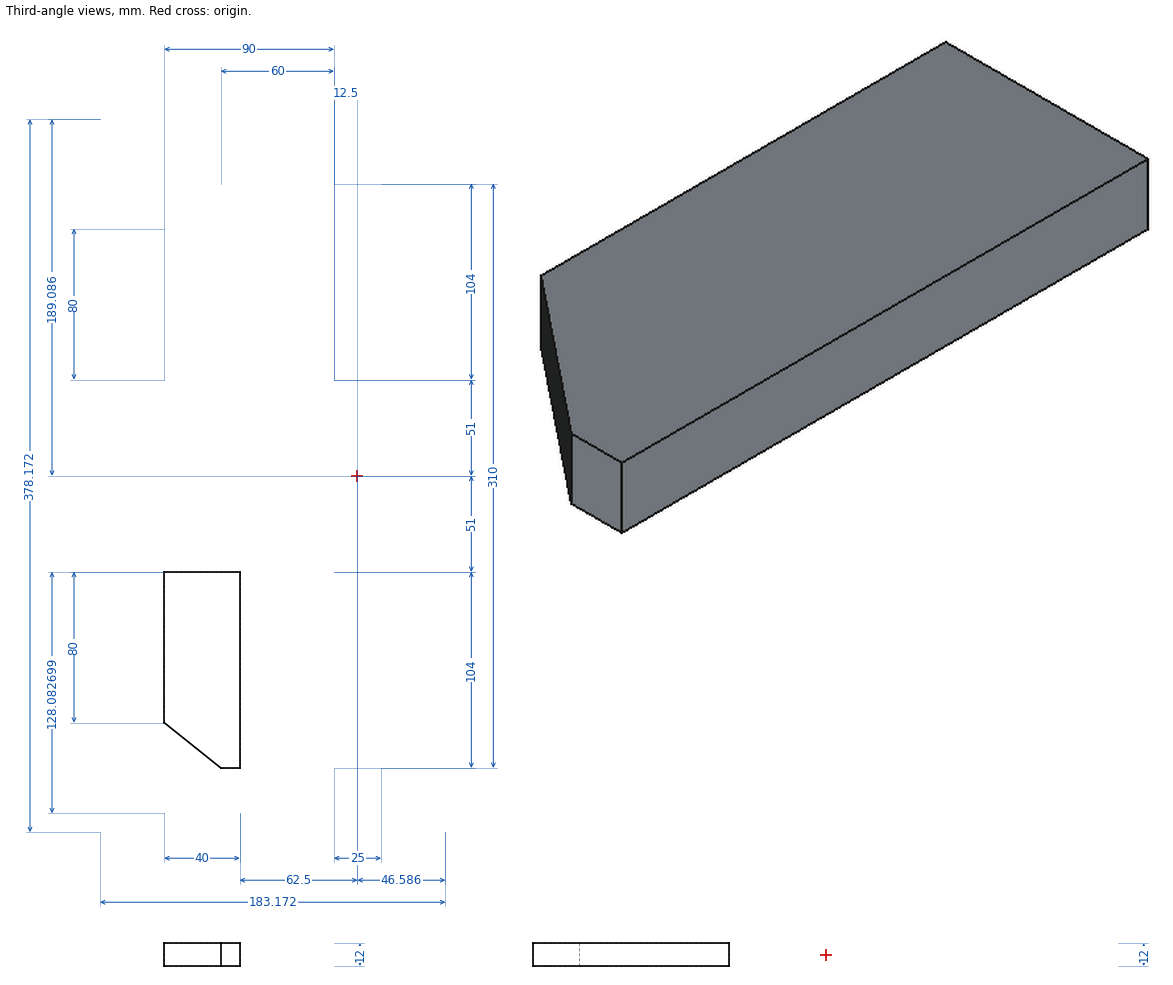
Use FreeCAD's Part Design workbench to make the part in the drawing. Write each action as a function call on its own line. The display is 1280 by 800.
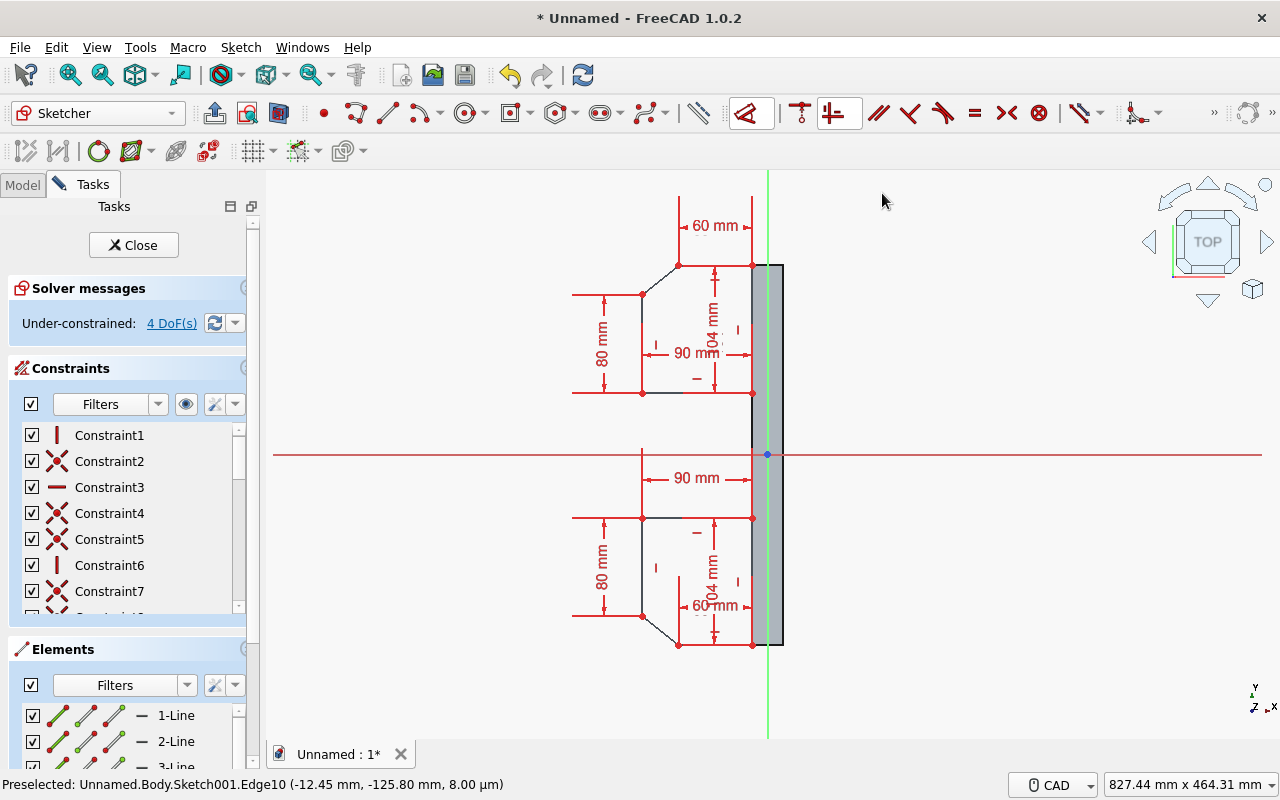
click(752, 393)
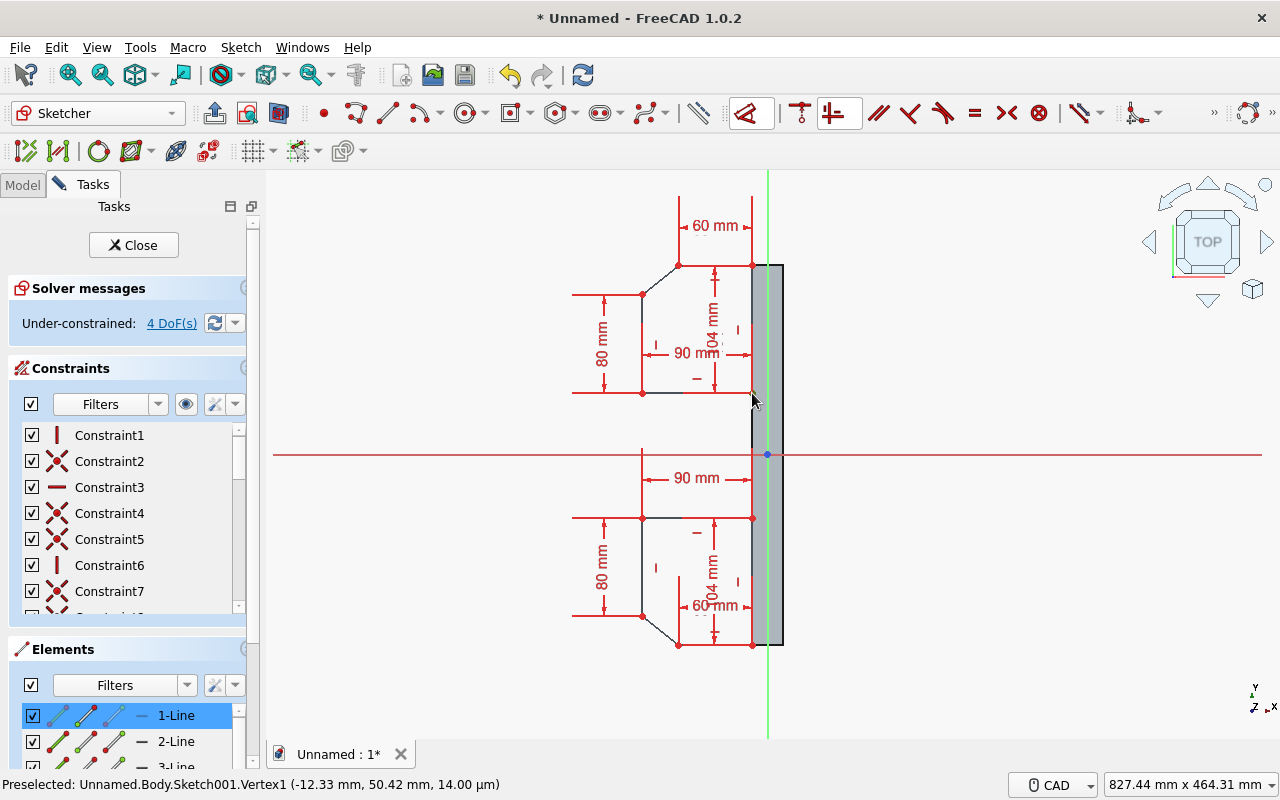
click(768, 114)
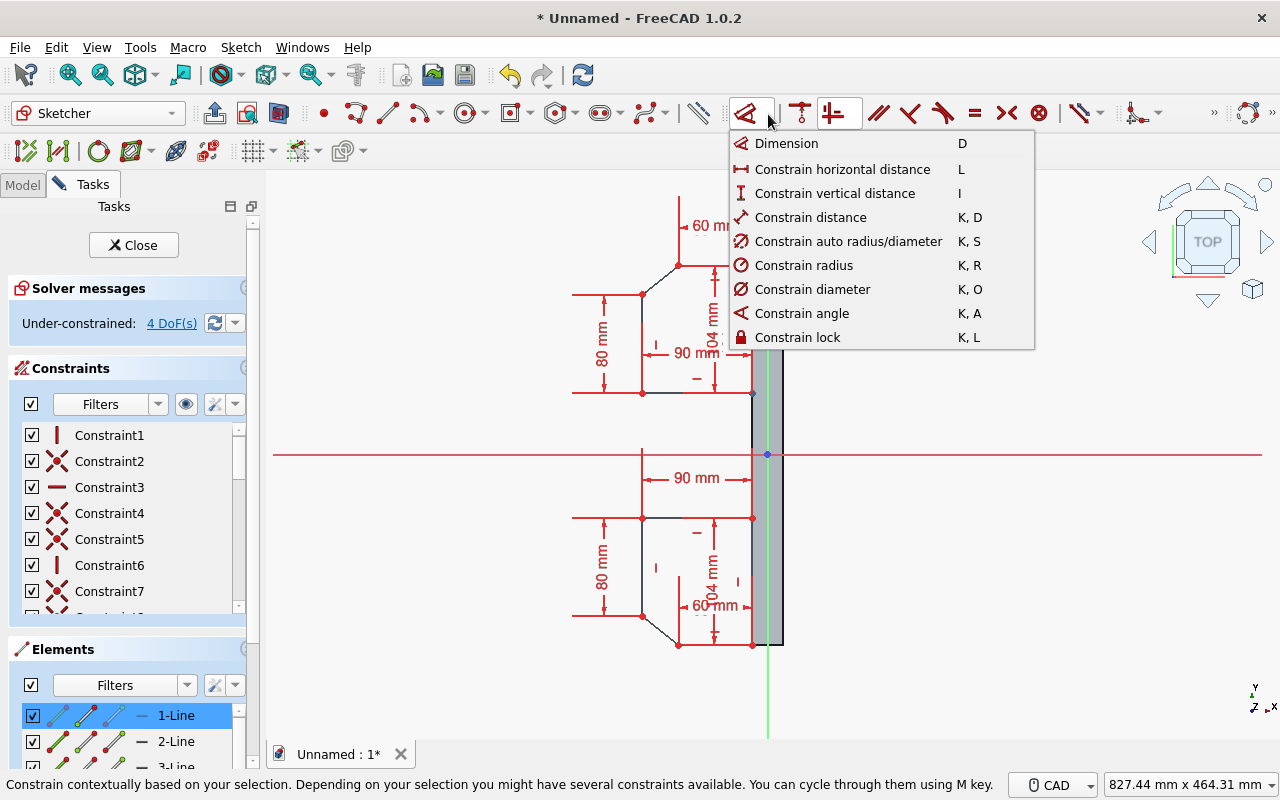
click(882, 193)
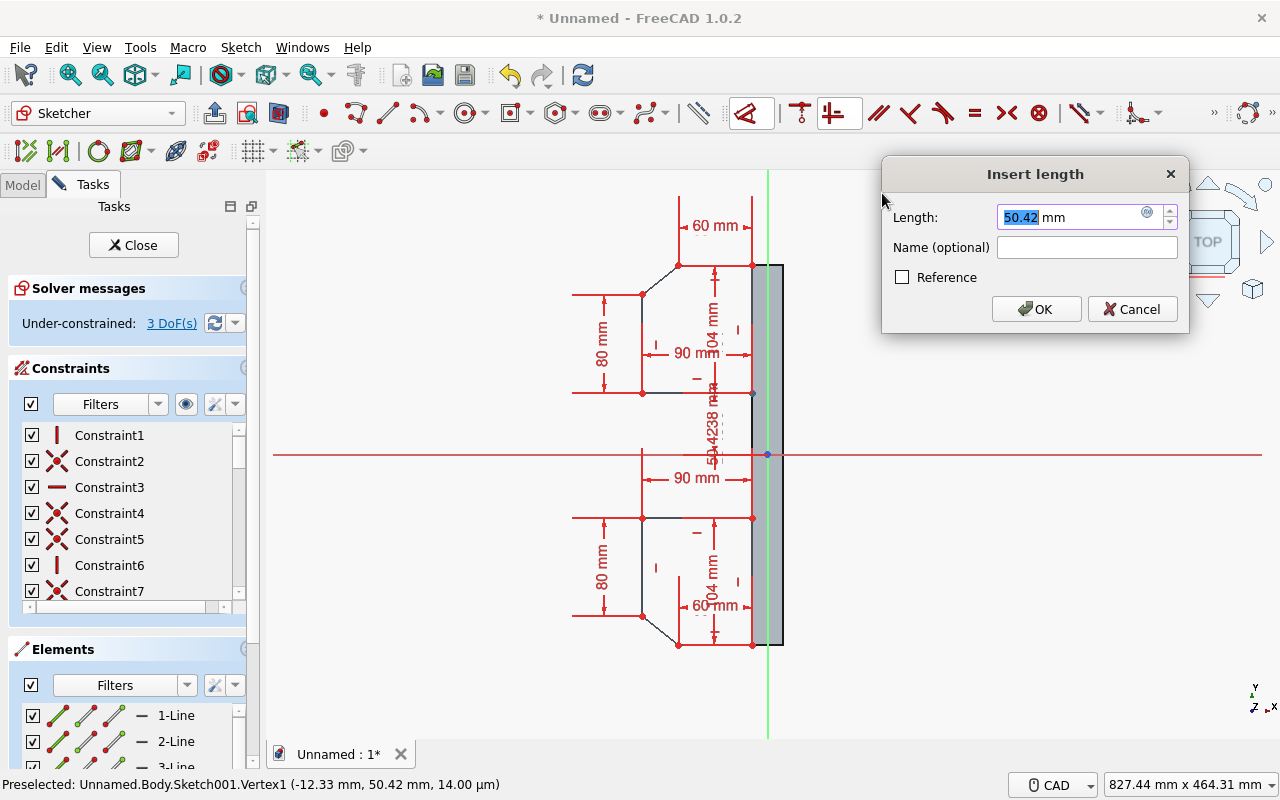
text(51)
key(Return)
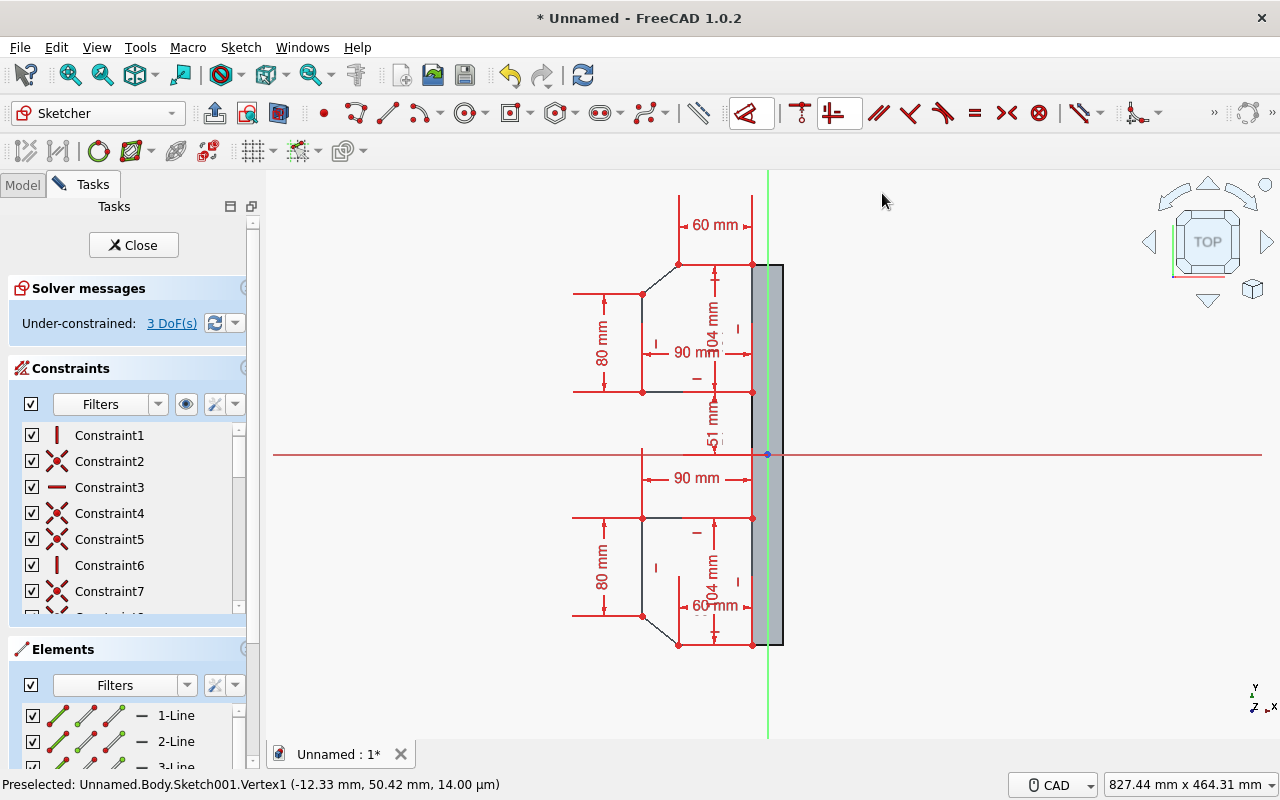
click(752, 518)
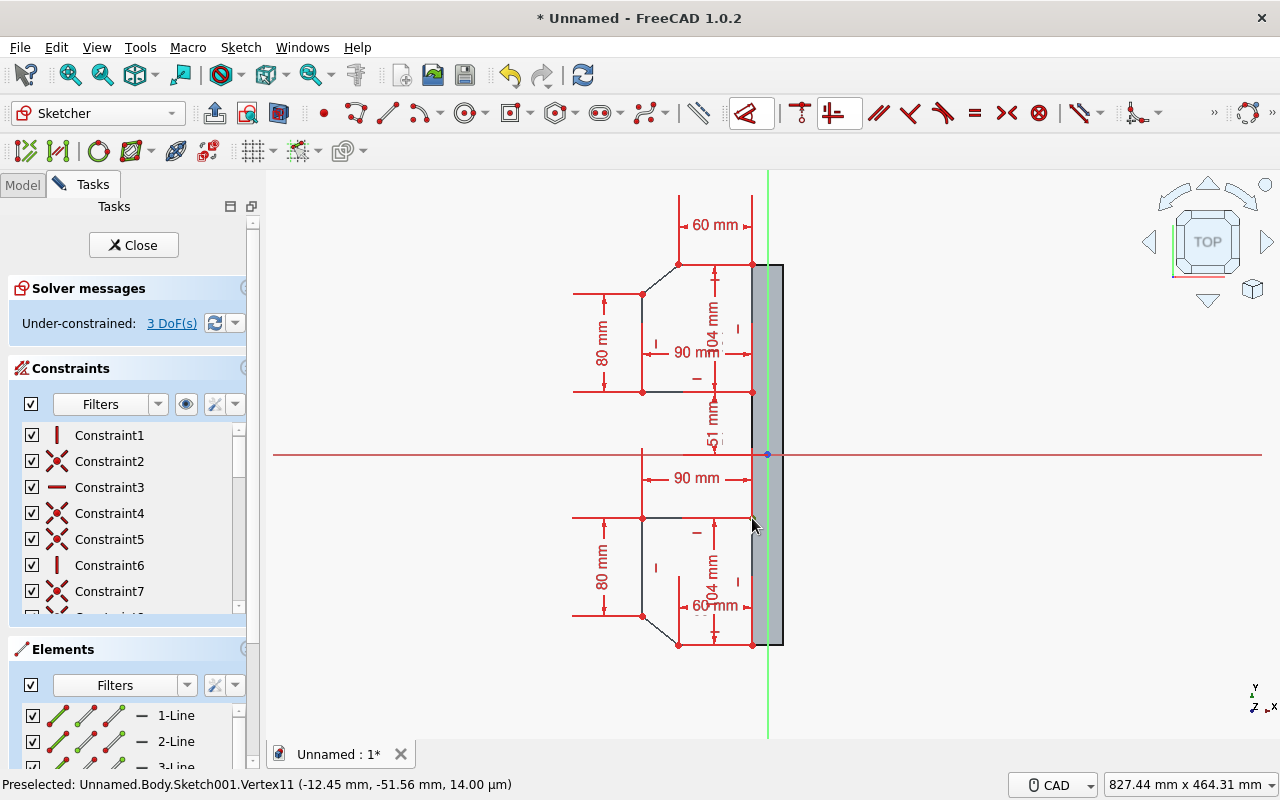
click(768, 114)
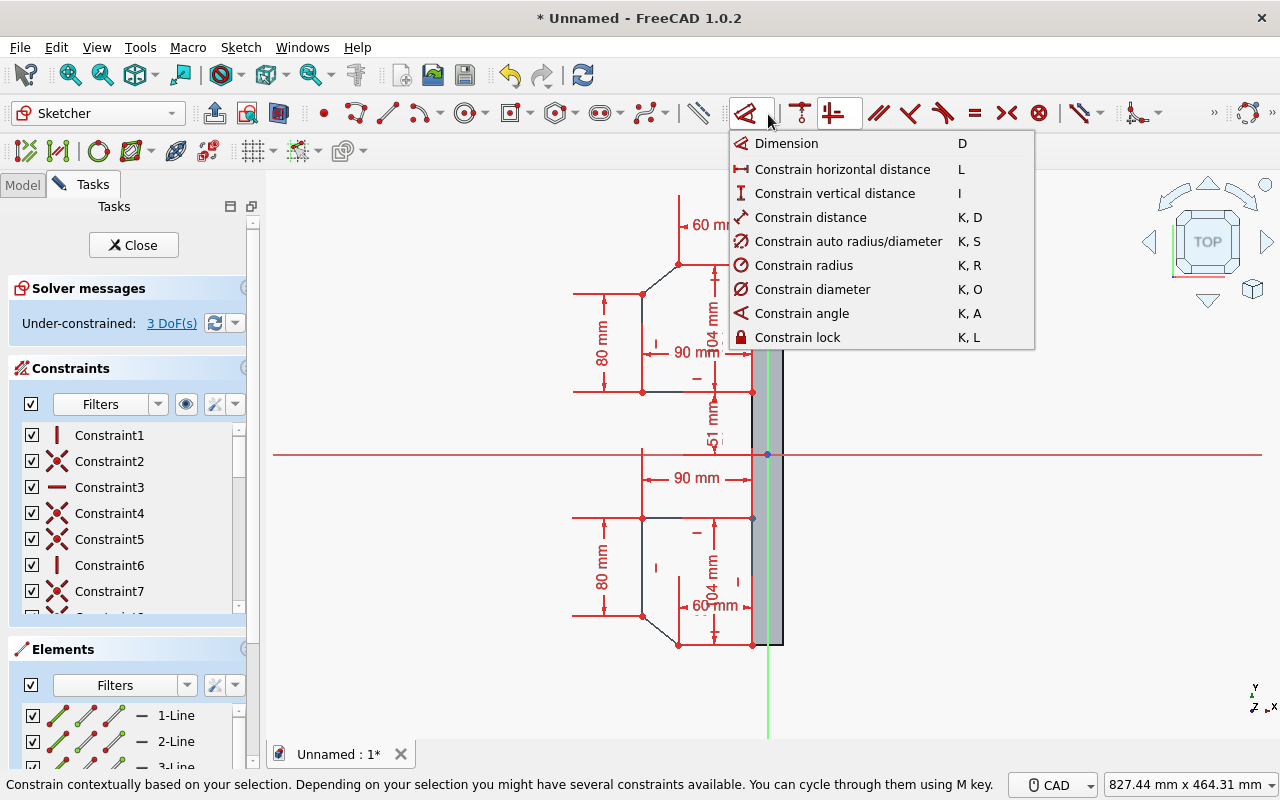
click(882, 193)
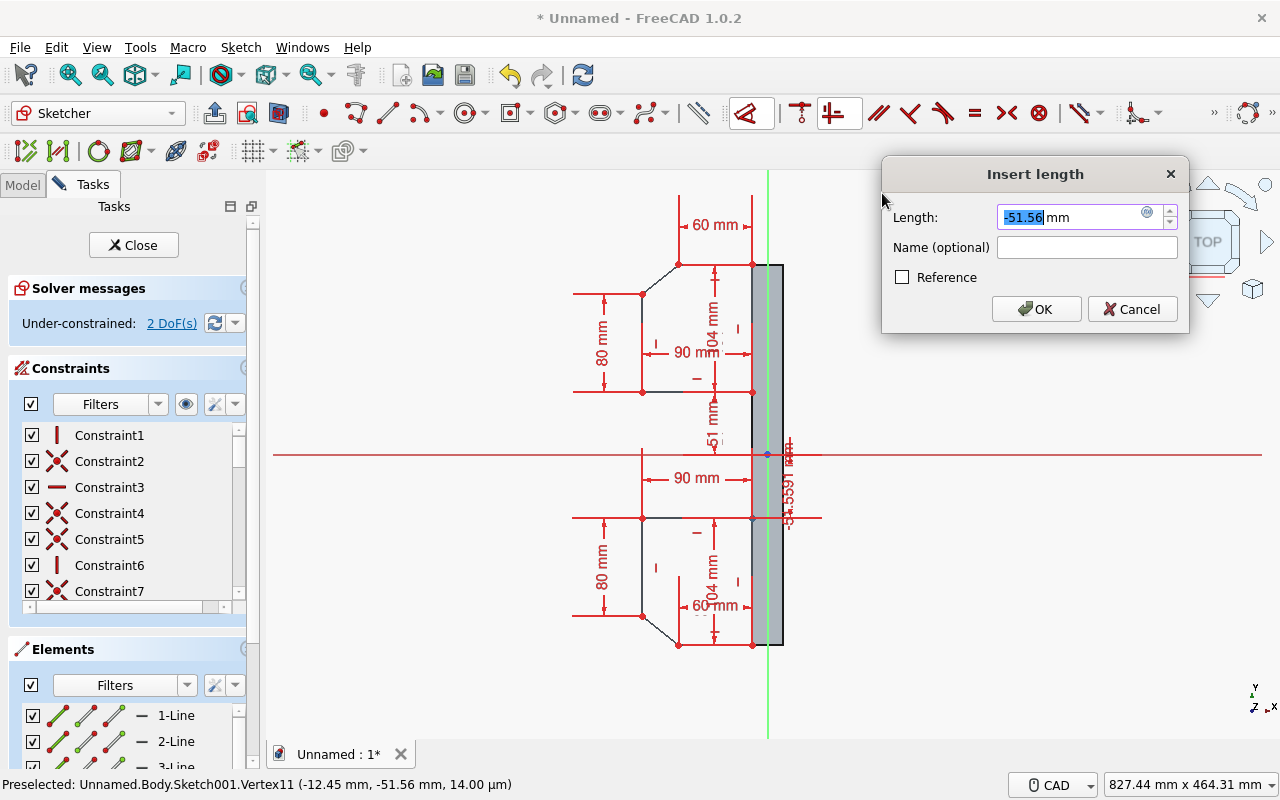
text(-51)
key(Return)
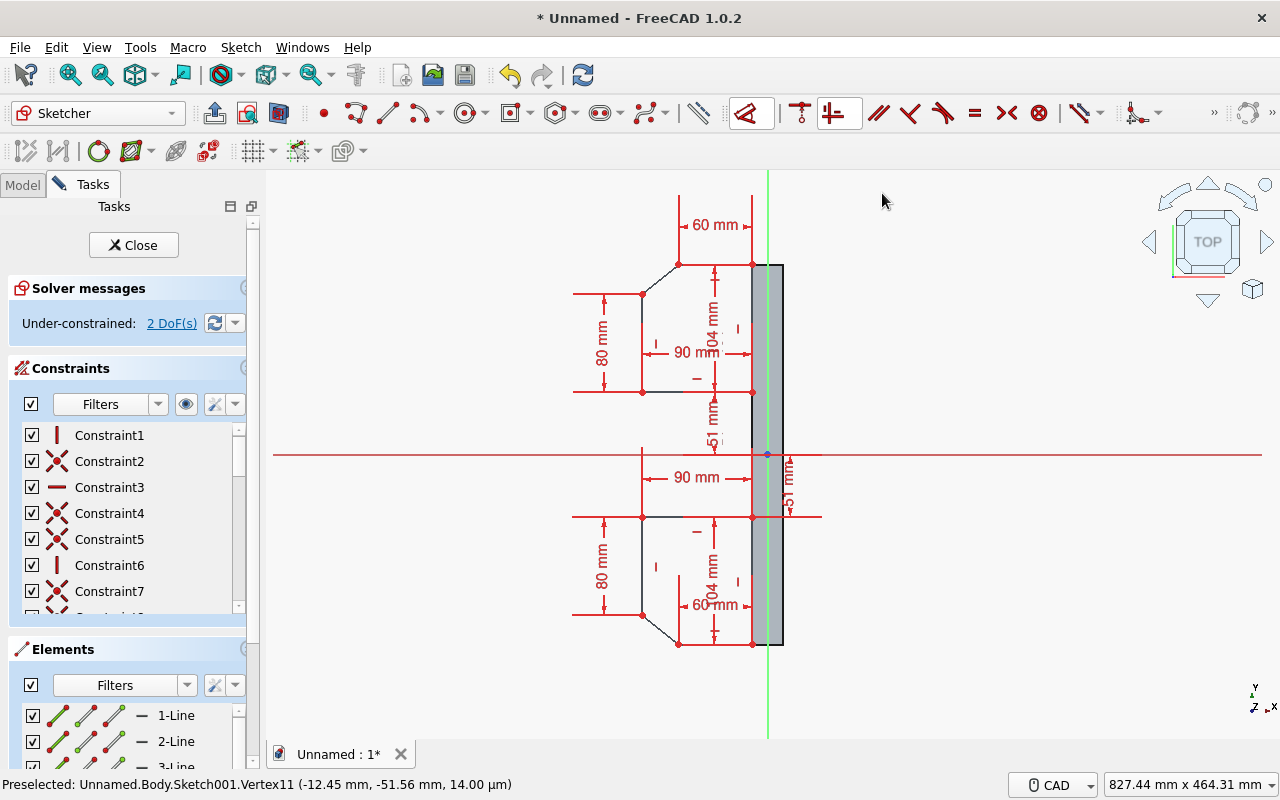
scroll(752, 392, up, 5)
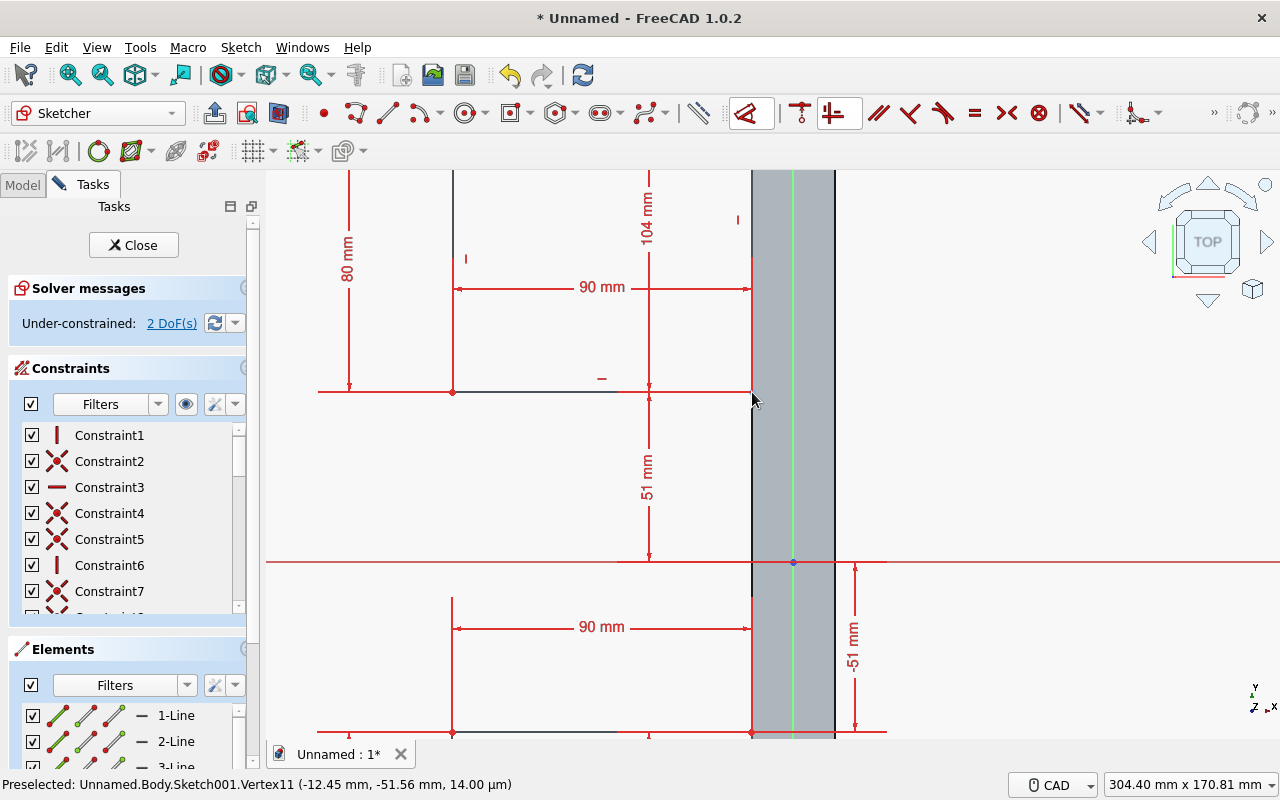
click(752, 392)